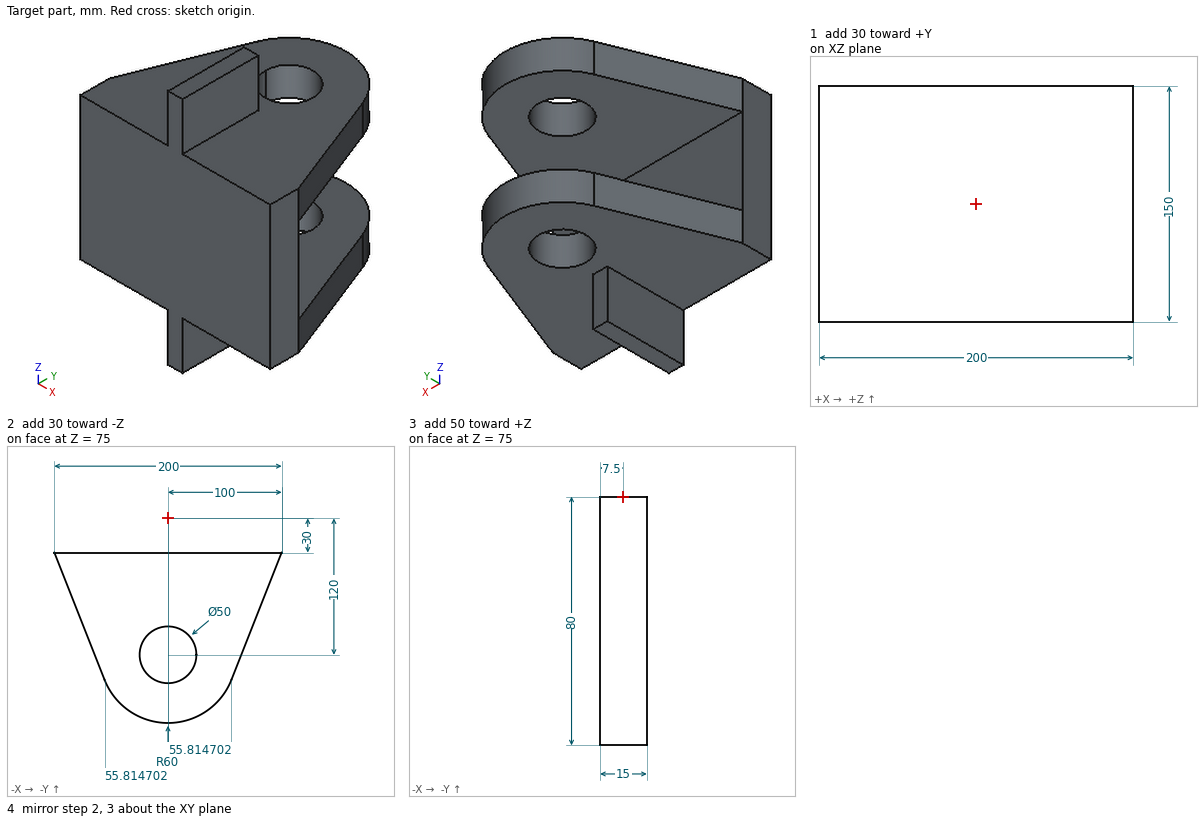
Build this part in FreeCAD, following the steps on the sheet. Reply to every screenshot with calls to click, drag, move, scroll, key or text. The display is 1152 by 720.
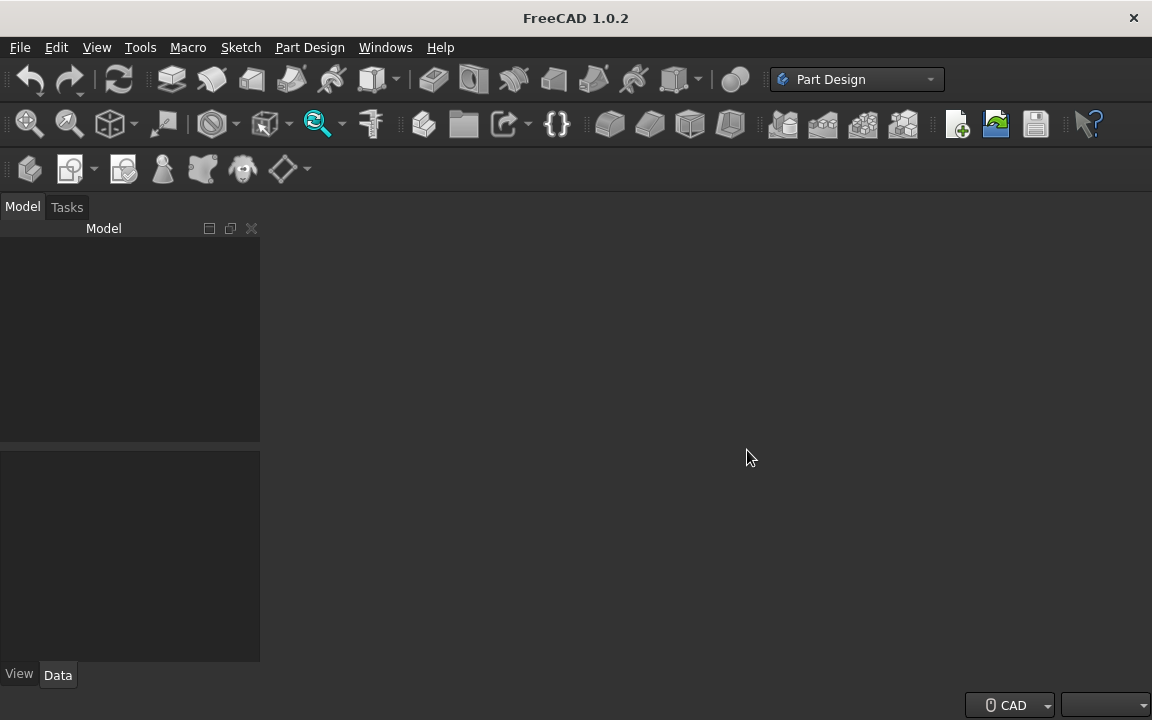
key(ctrl+n)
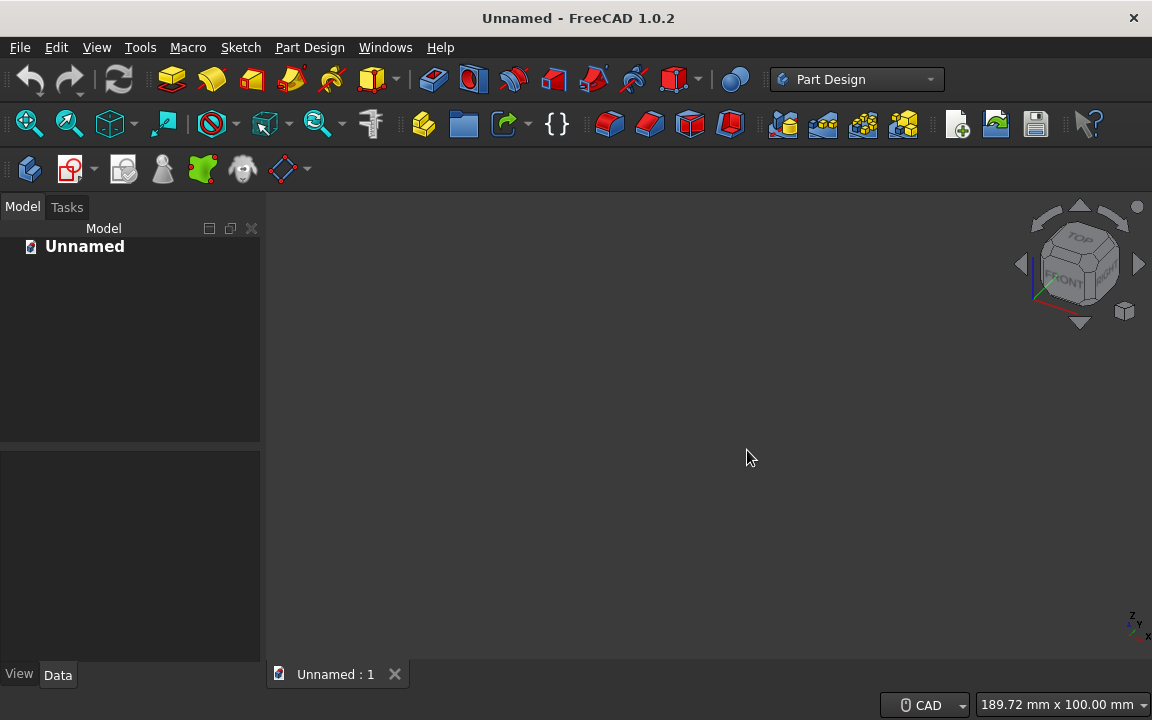
click(70, 170)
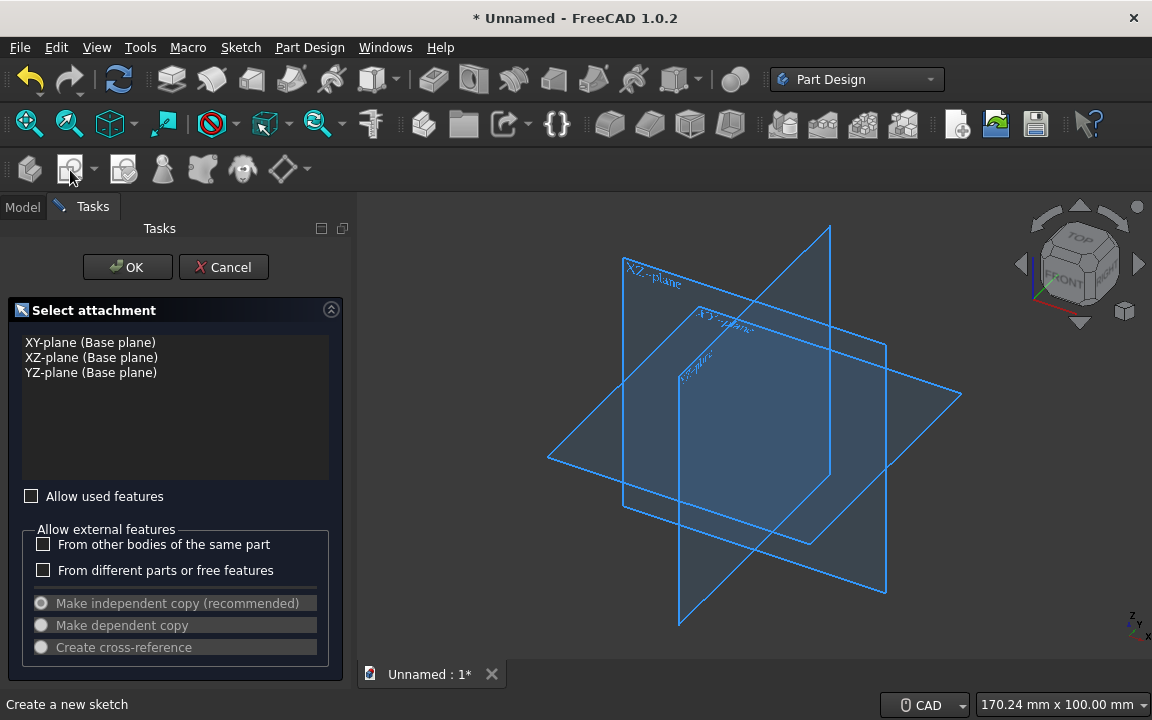
click(82, 358)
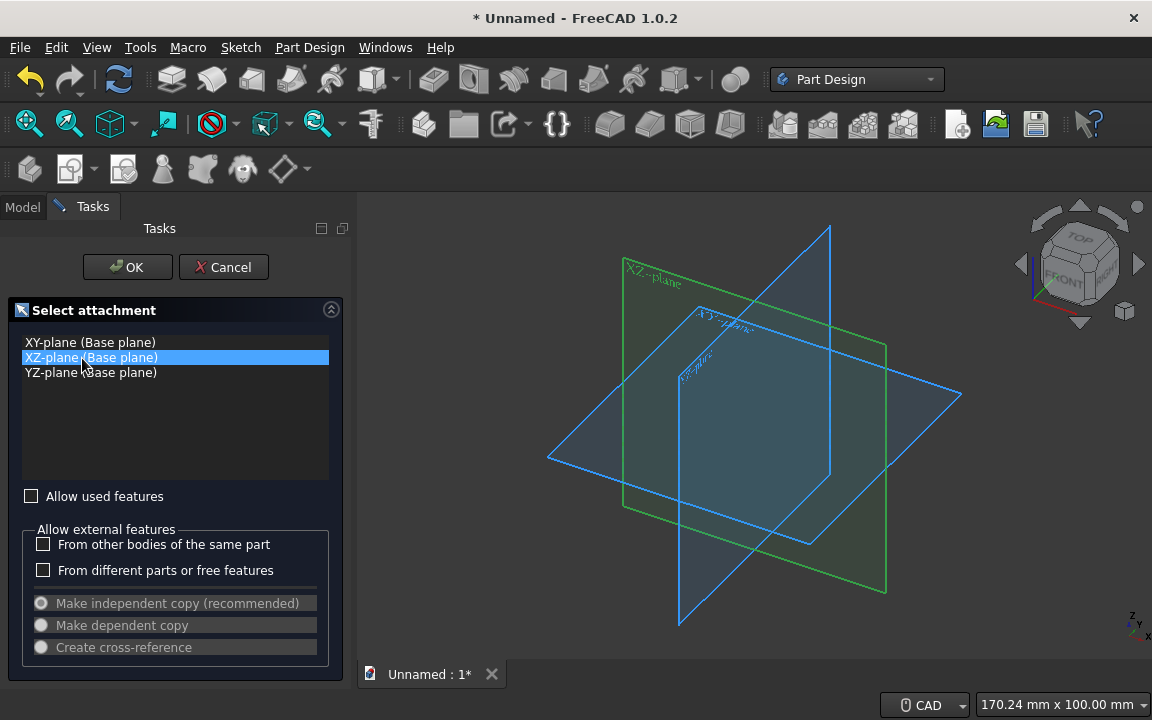
click(128, 267)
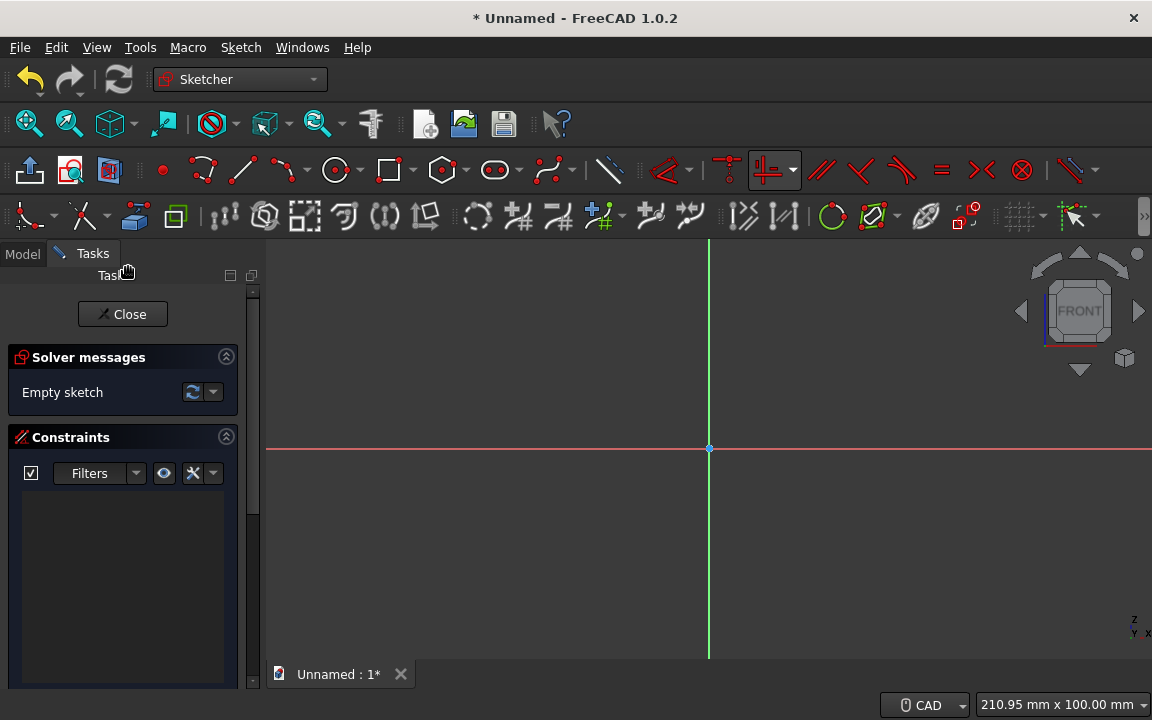
scroll(585, 449, down, 4)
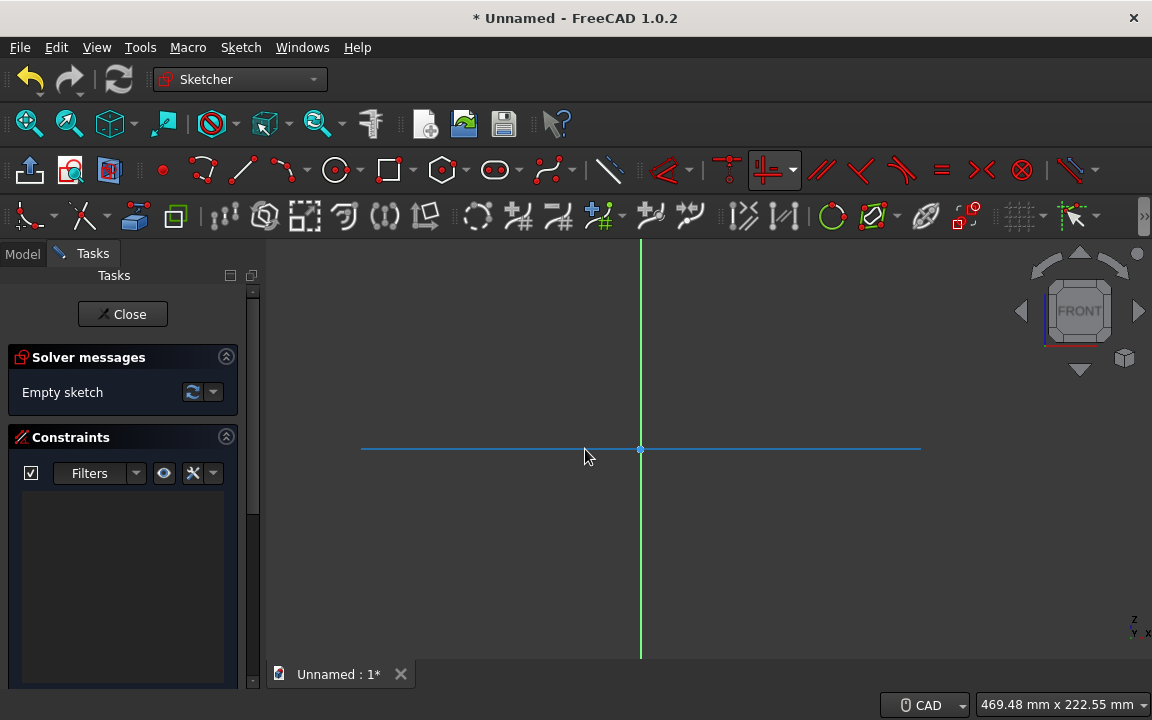
click(416, 170)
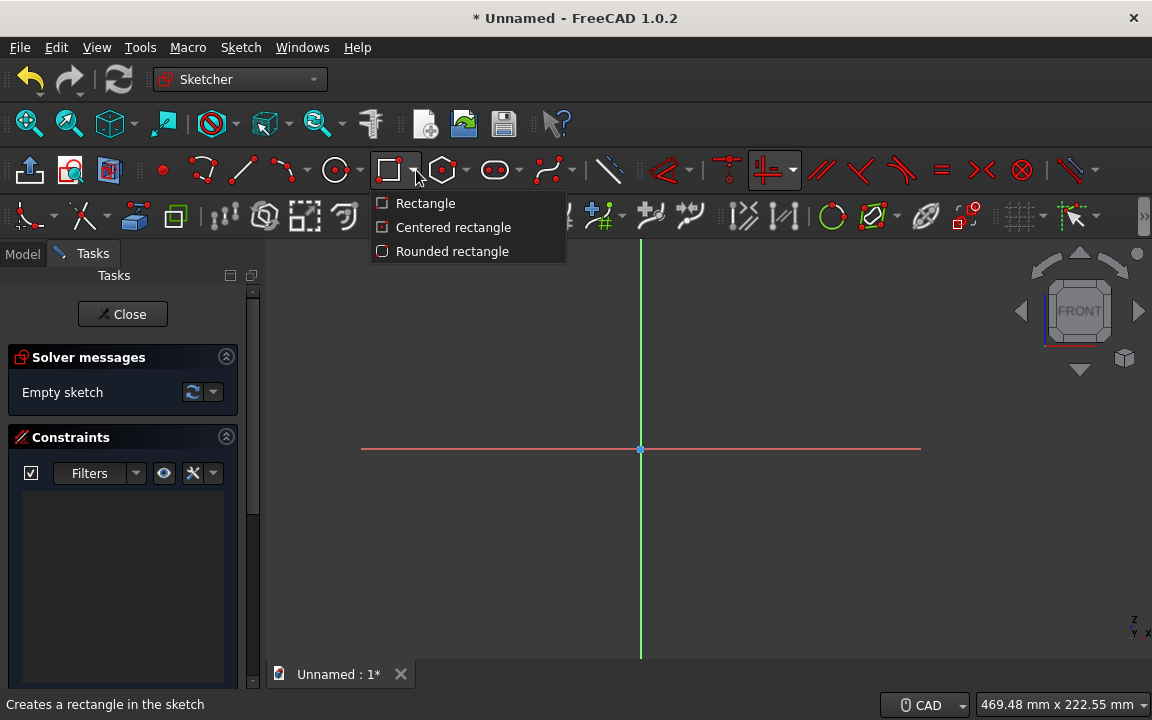
click(468, 227)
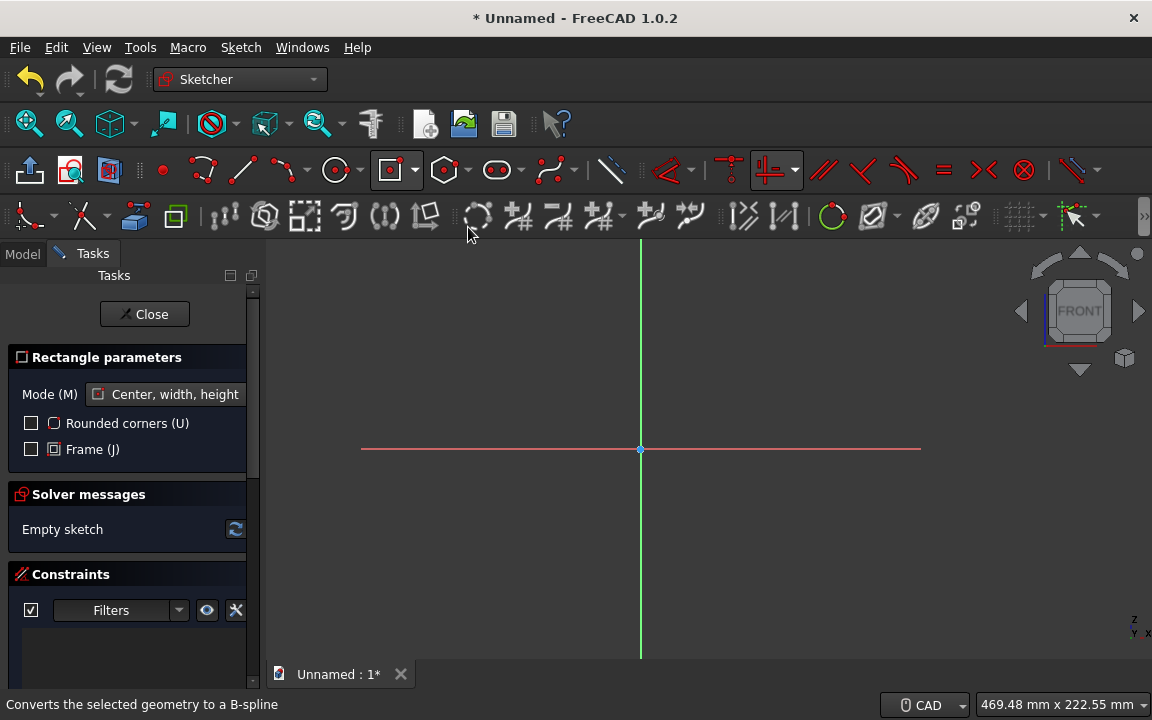
click(641, 449)
click(830, 308)
key(Escape)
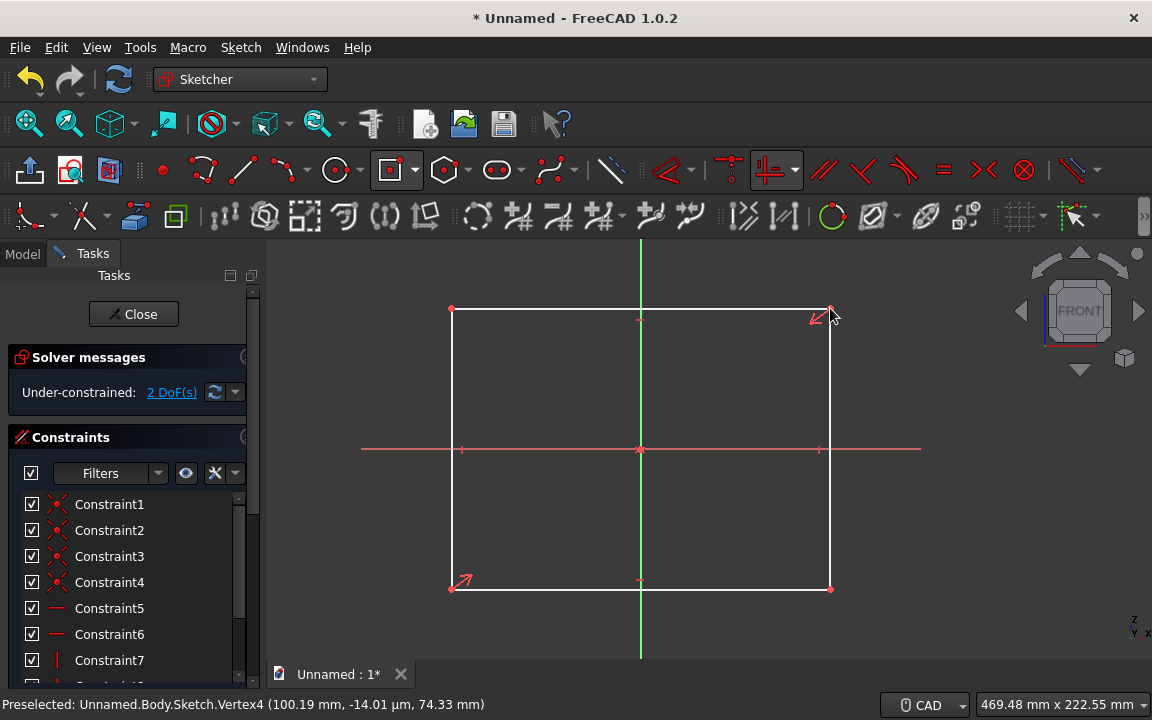
key(d)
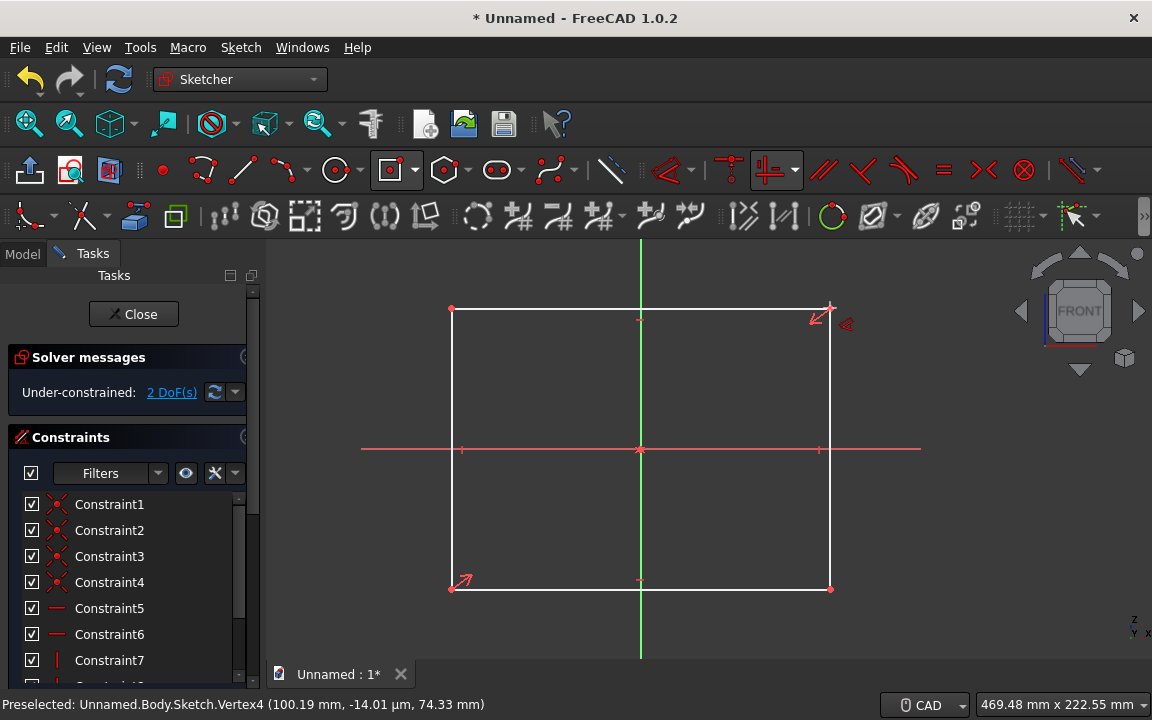
click(565, 590)
click(554, 624)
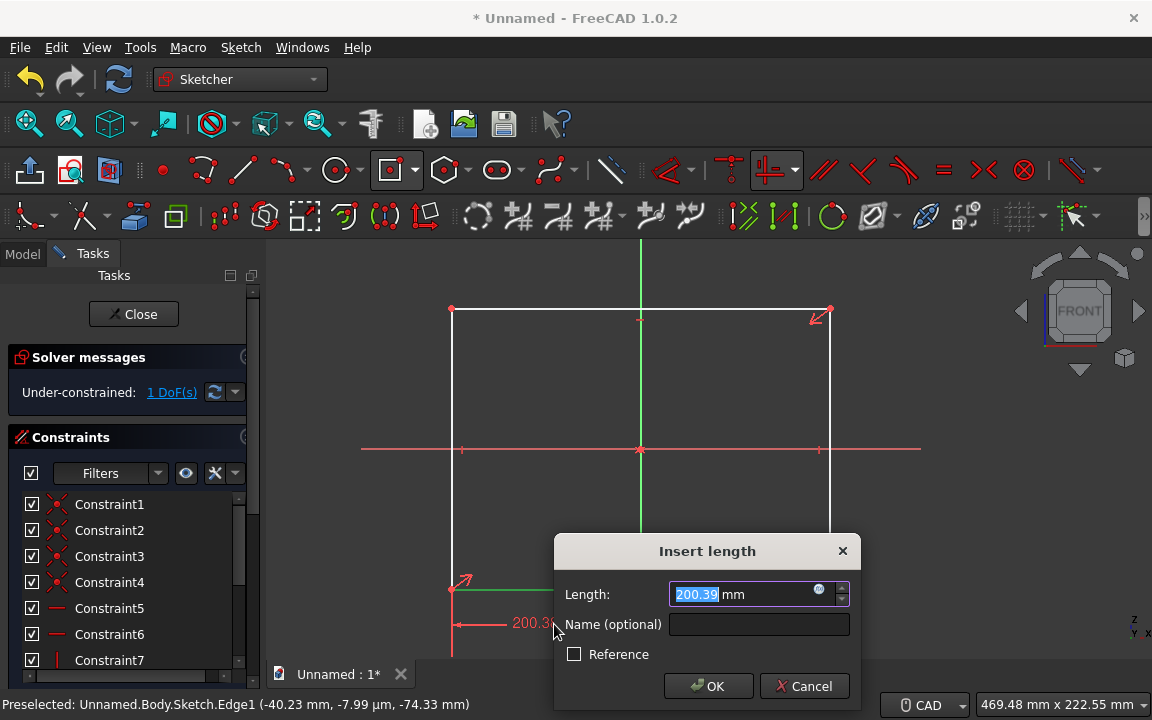
text(200)
key(Return)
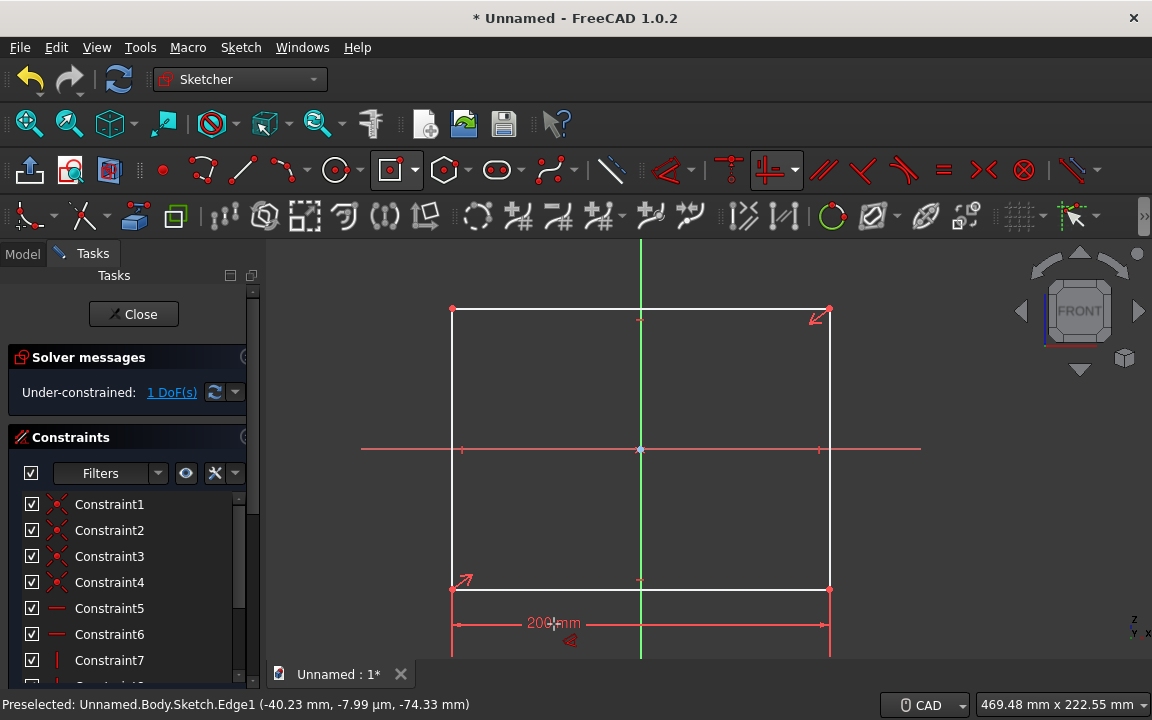
click(830, 505)
click(864, 385)